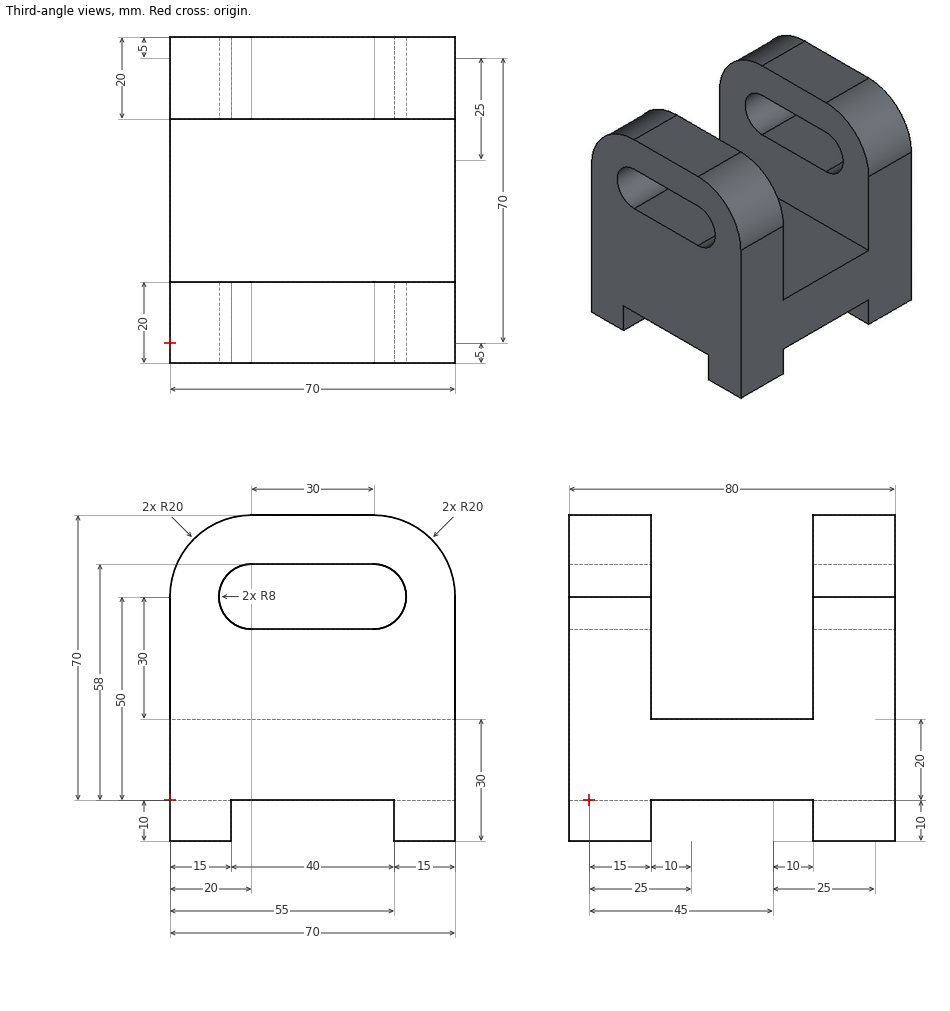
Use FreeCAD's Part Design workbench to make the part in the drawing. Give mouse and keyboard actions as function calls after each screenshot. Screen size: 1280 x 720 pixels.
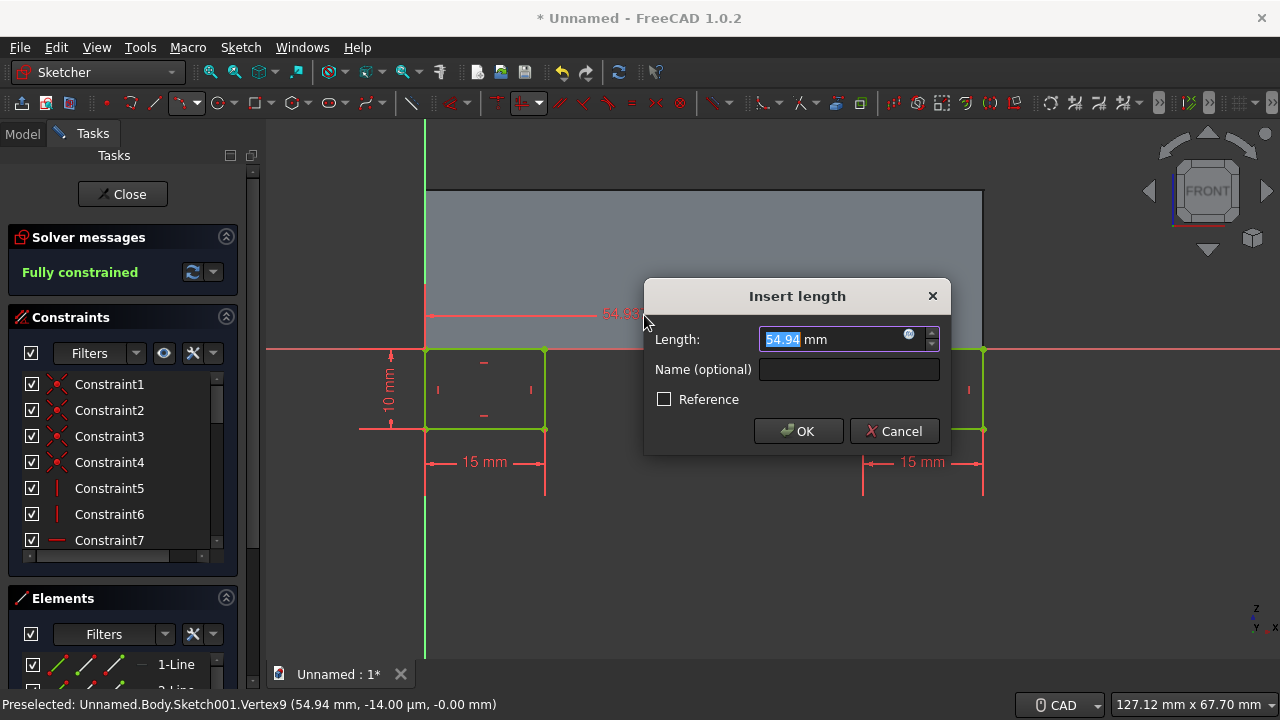
text(55)
key(Return)
key(Escape)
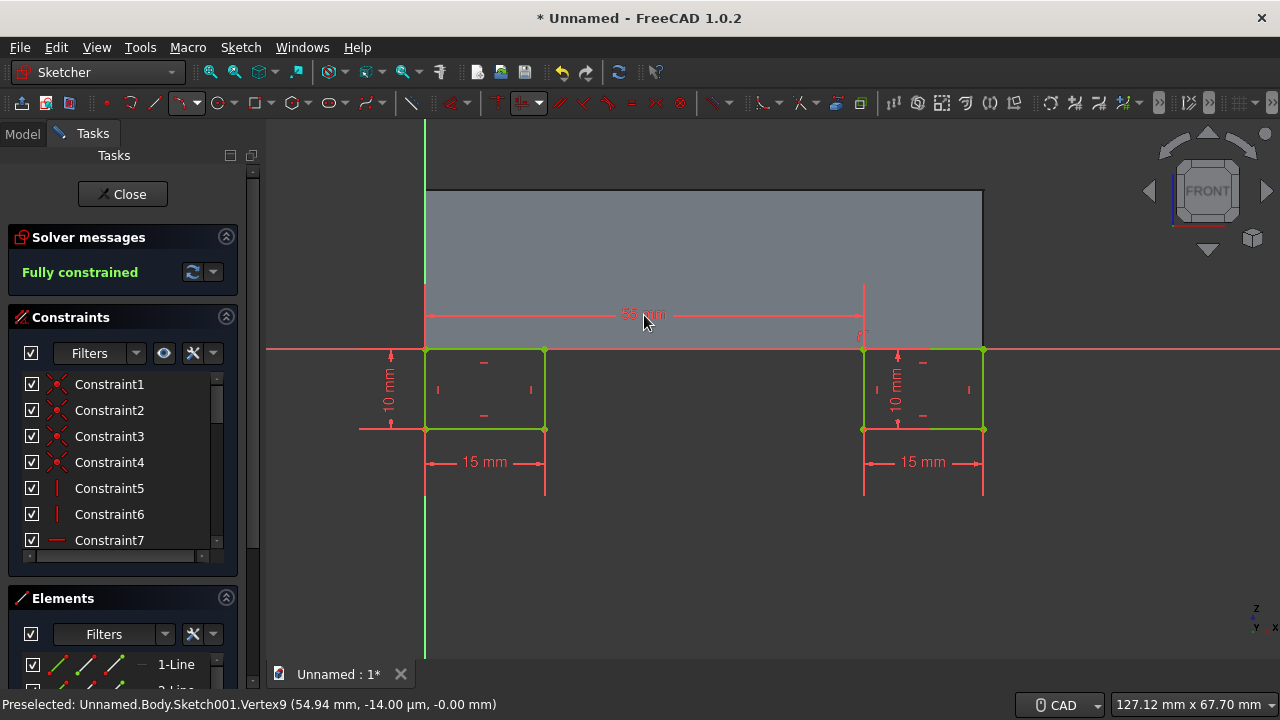
click(123, 194)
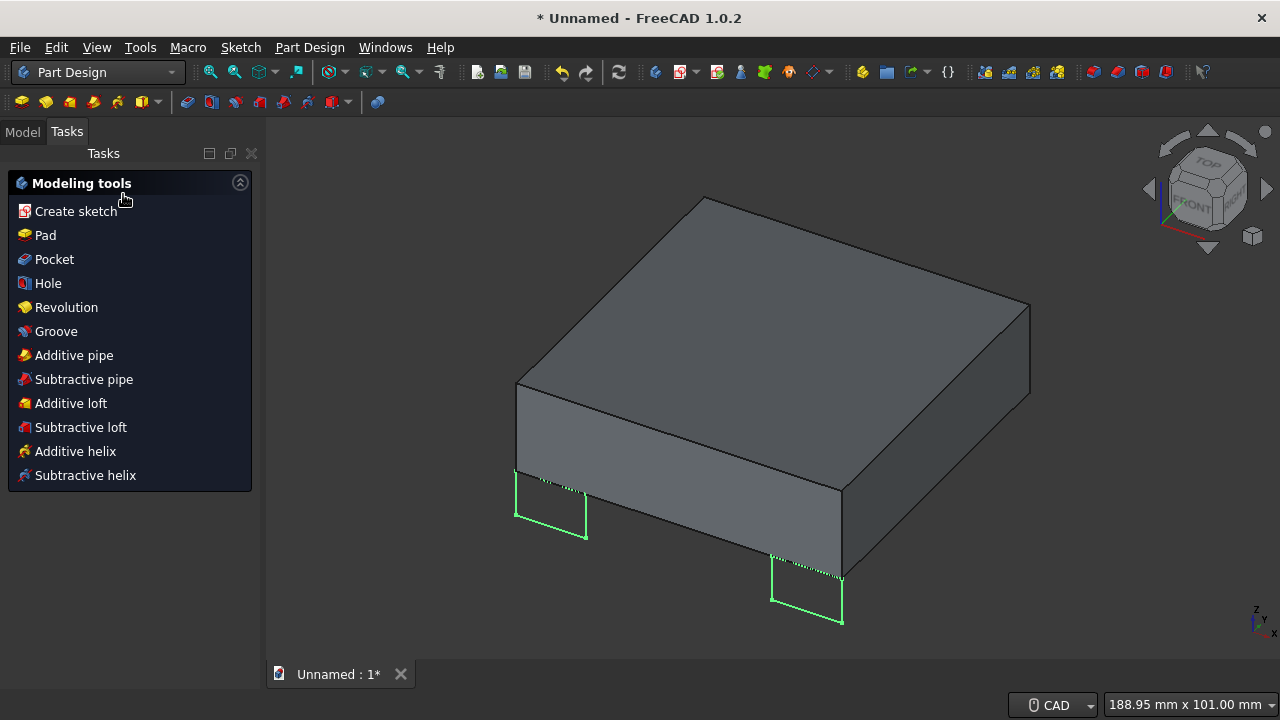
click(22, 102)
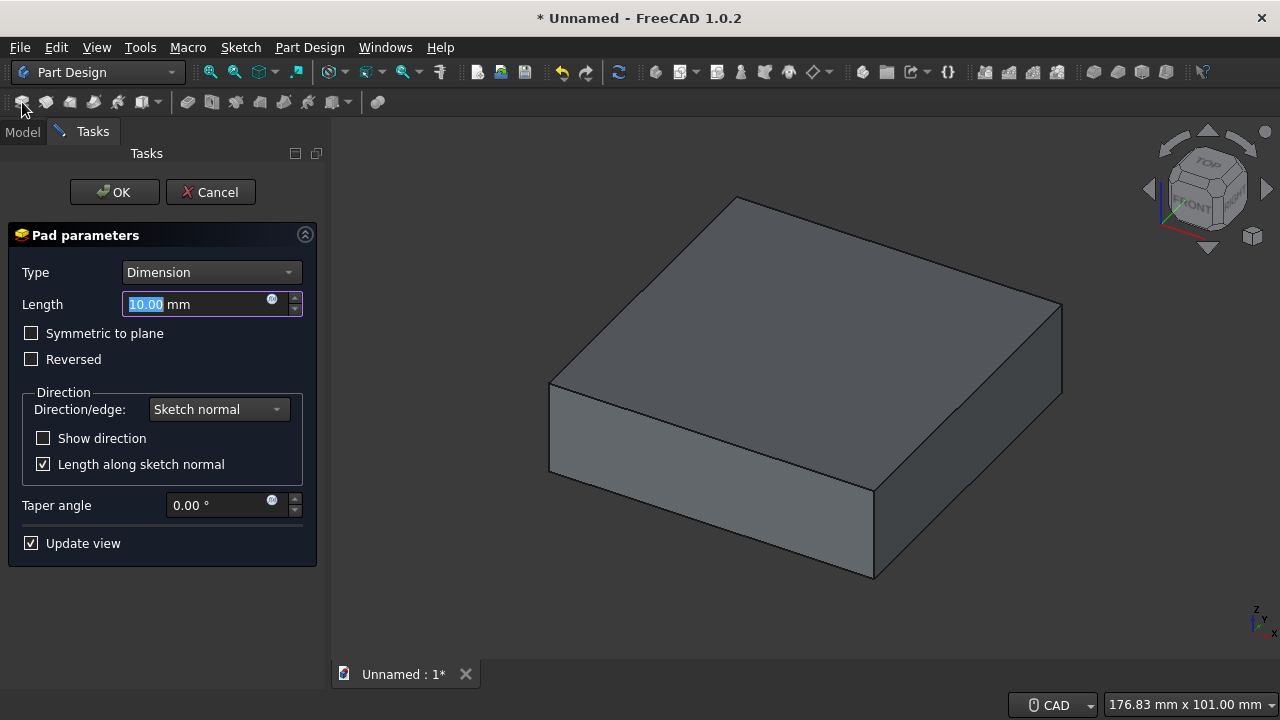
text(25)
key(Tab)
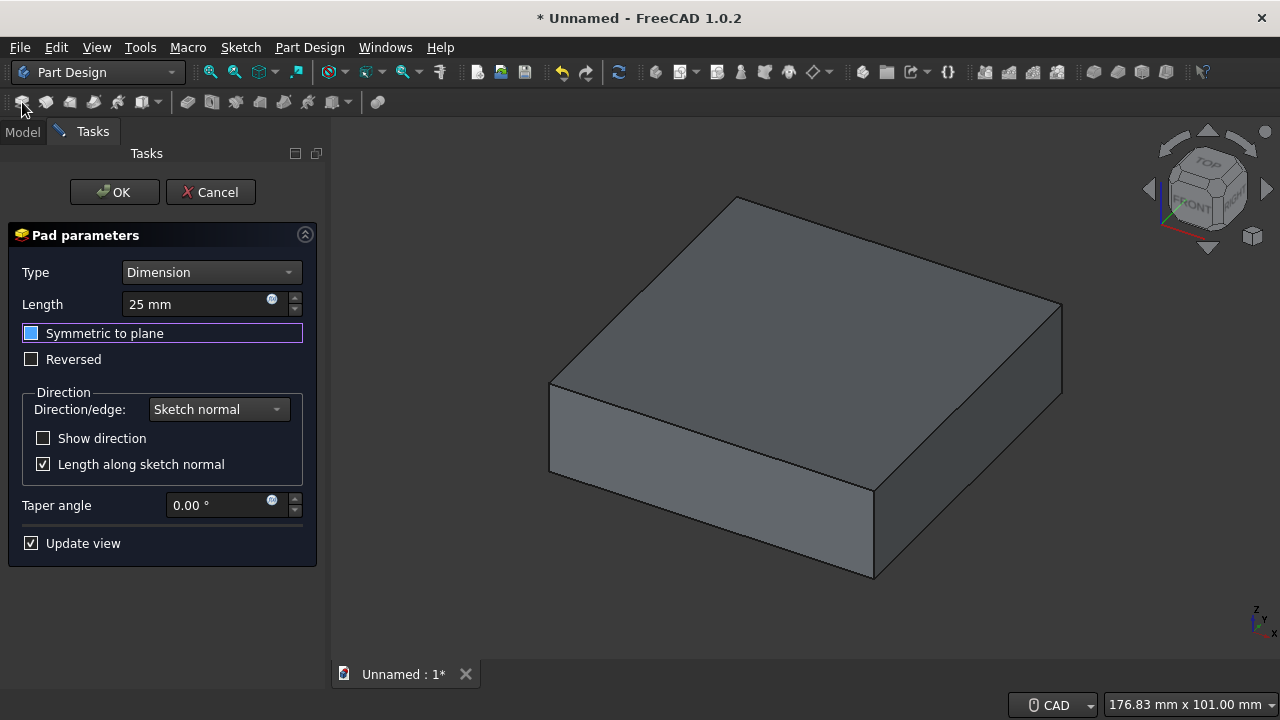
click(30, 359)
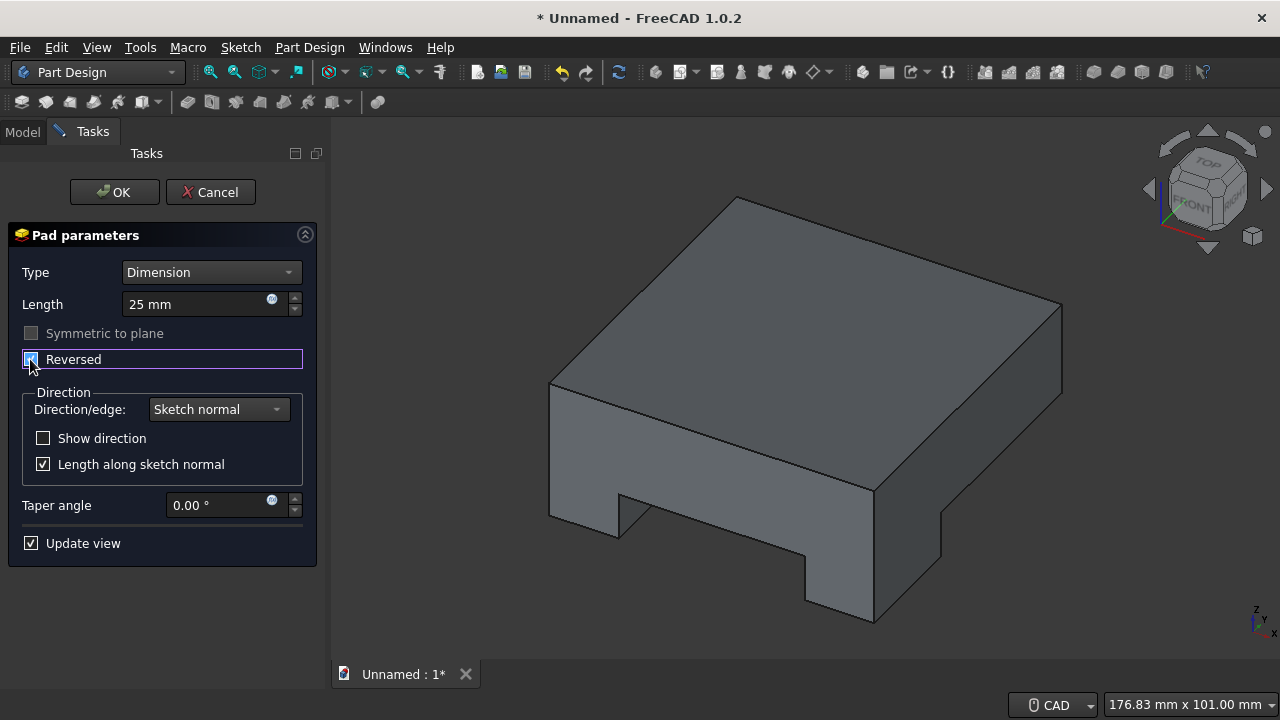
click(115, 192)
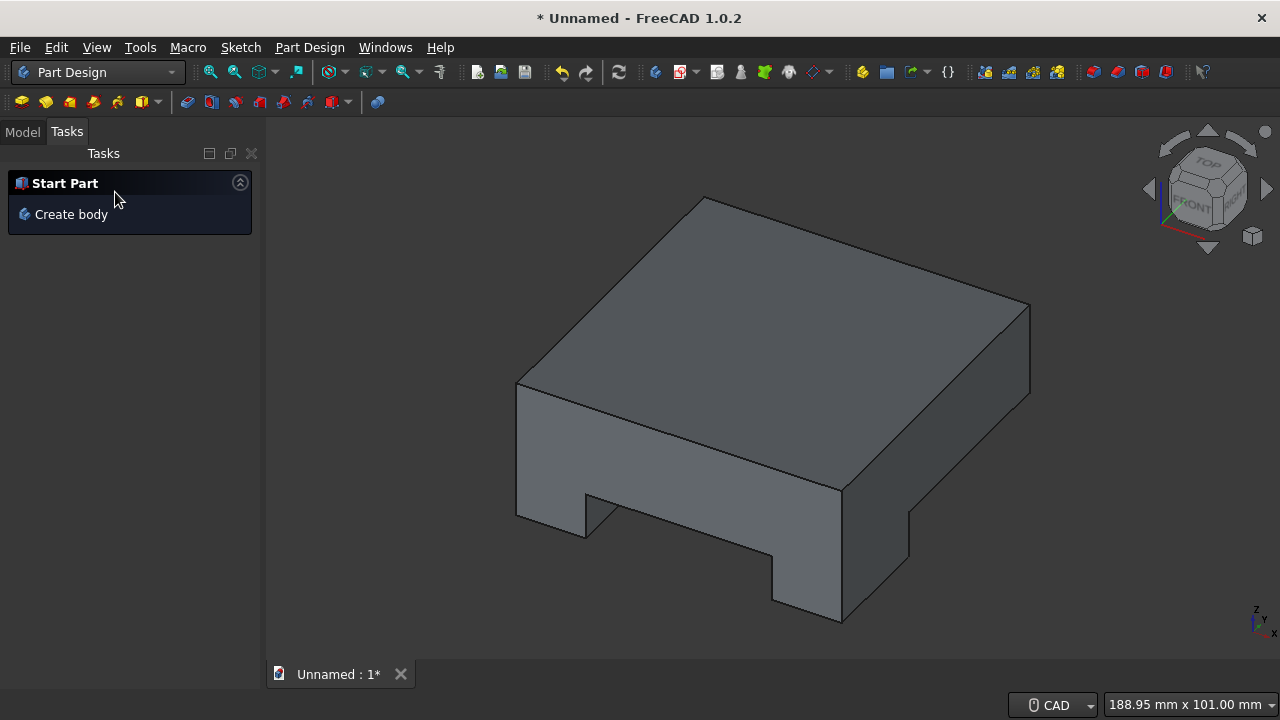
key(4)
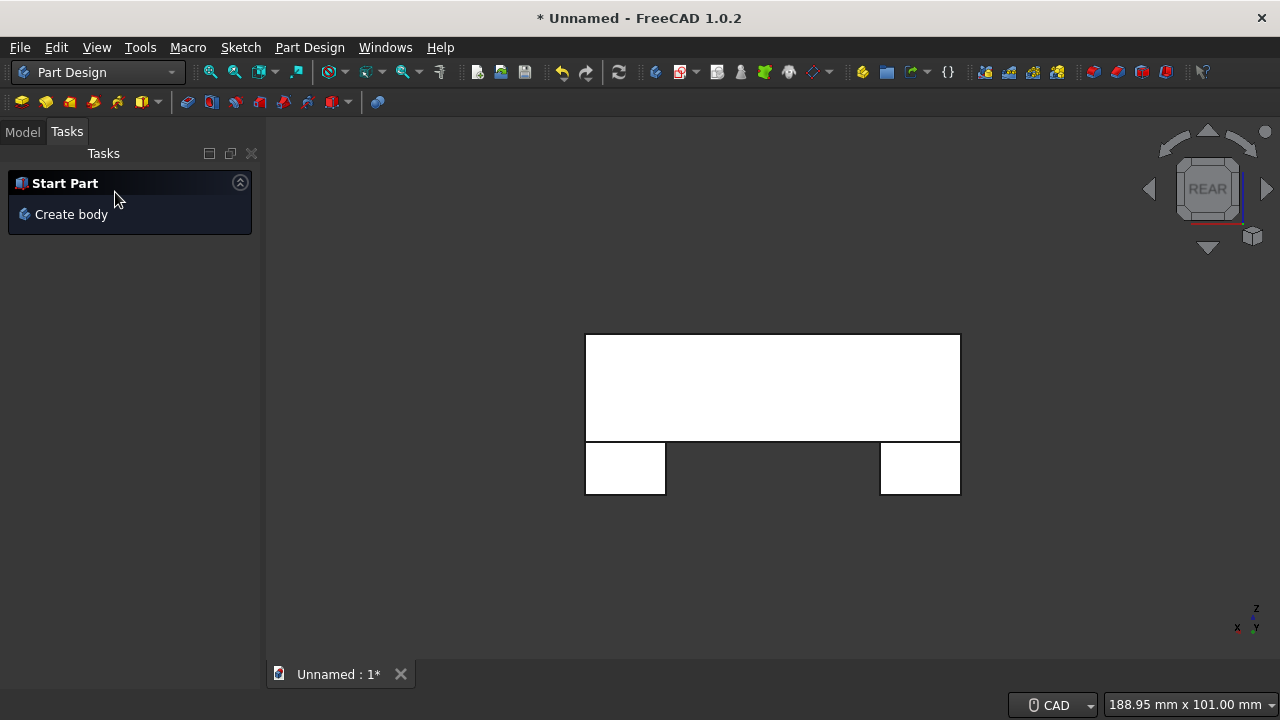
click(212, 72)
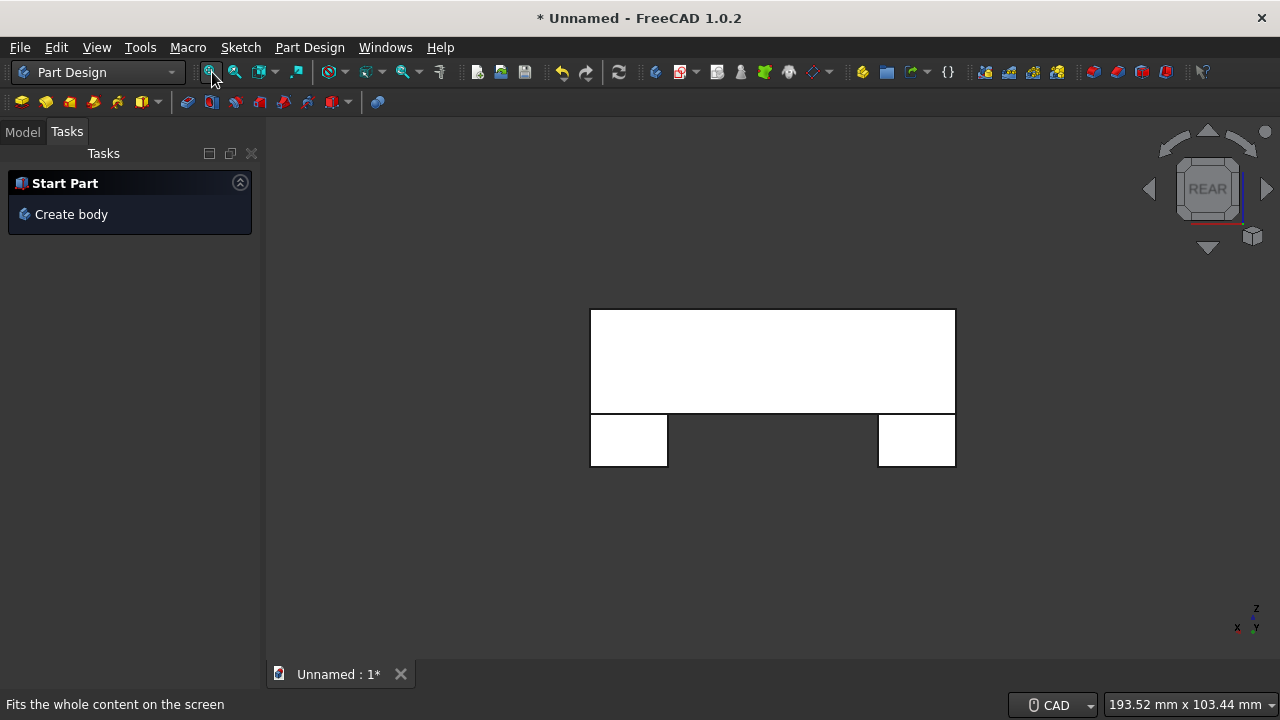
click(668, 361)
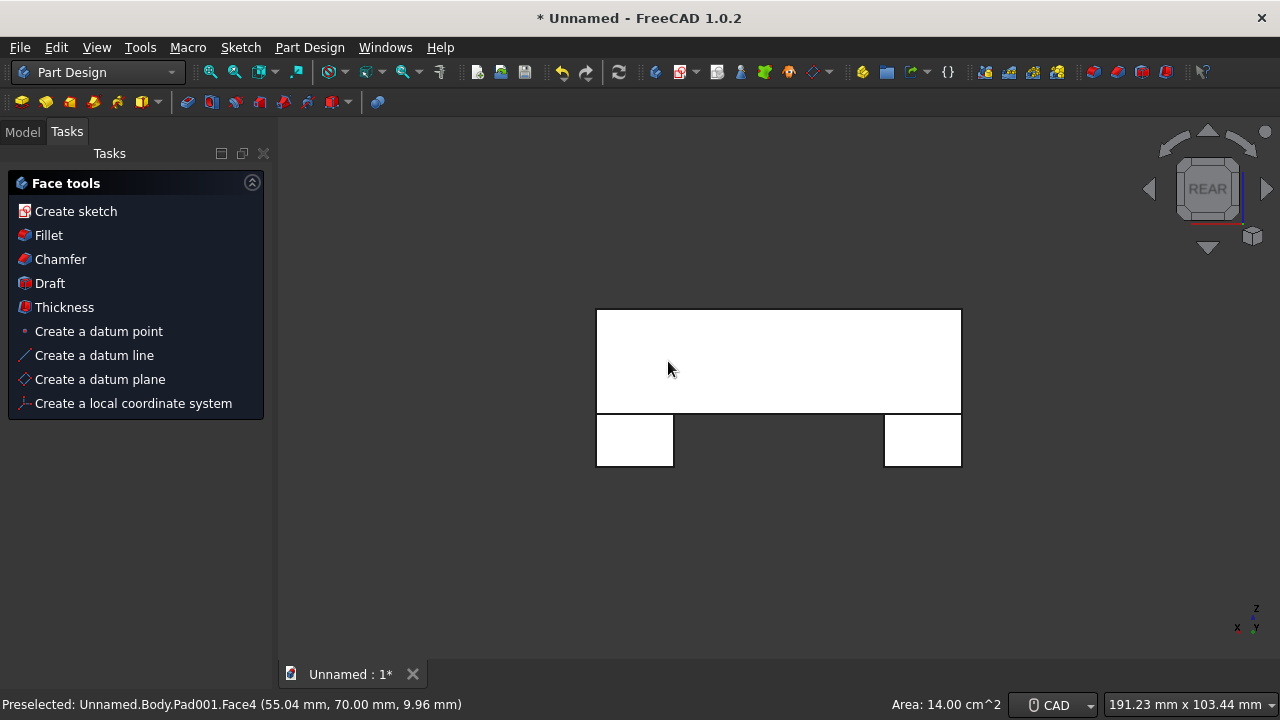
click(680, 72)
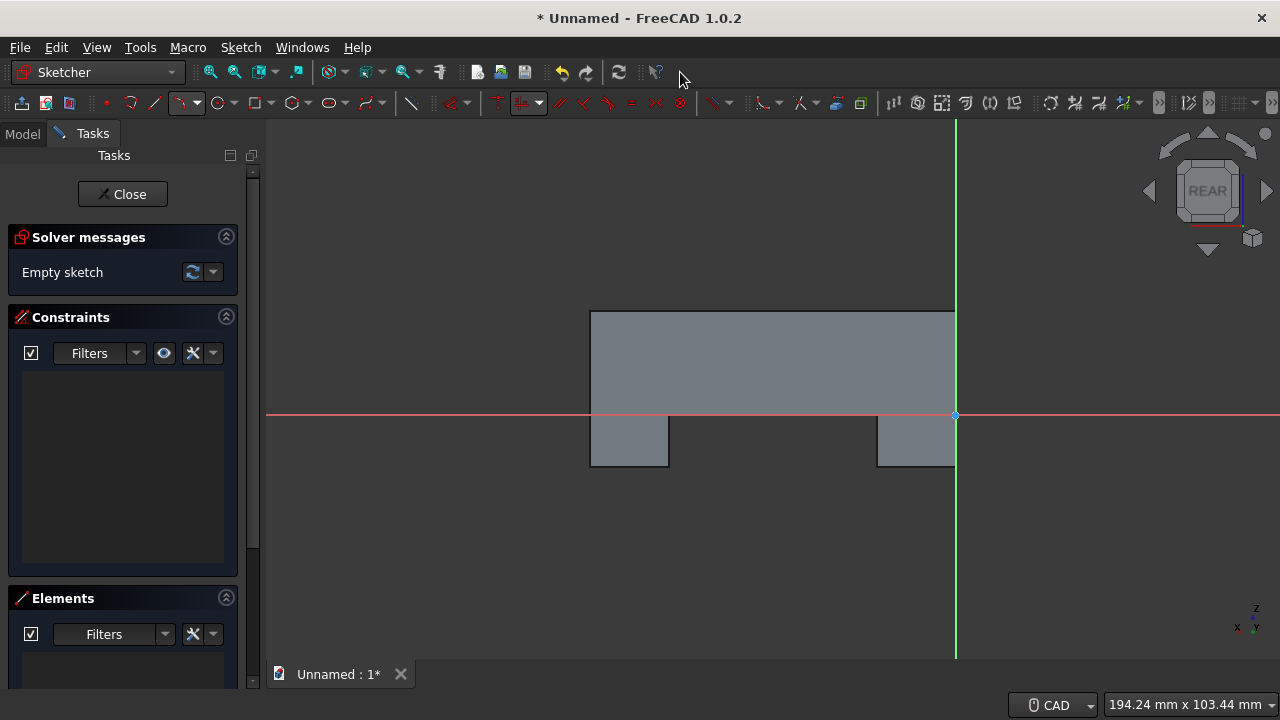
scroll(959, 452, up, 9)